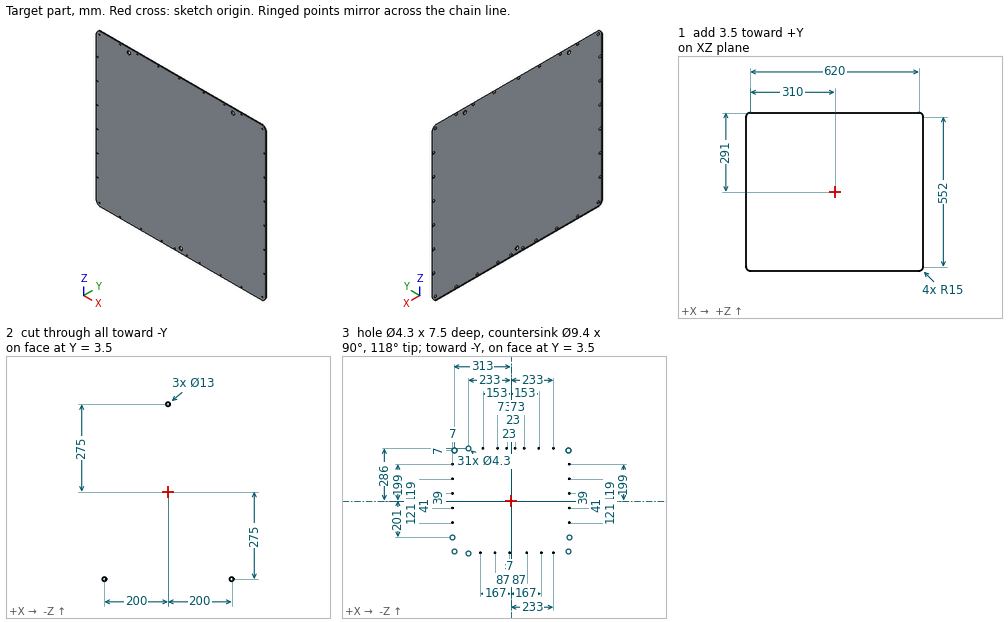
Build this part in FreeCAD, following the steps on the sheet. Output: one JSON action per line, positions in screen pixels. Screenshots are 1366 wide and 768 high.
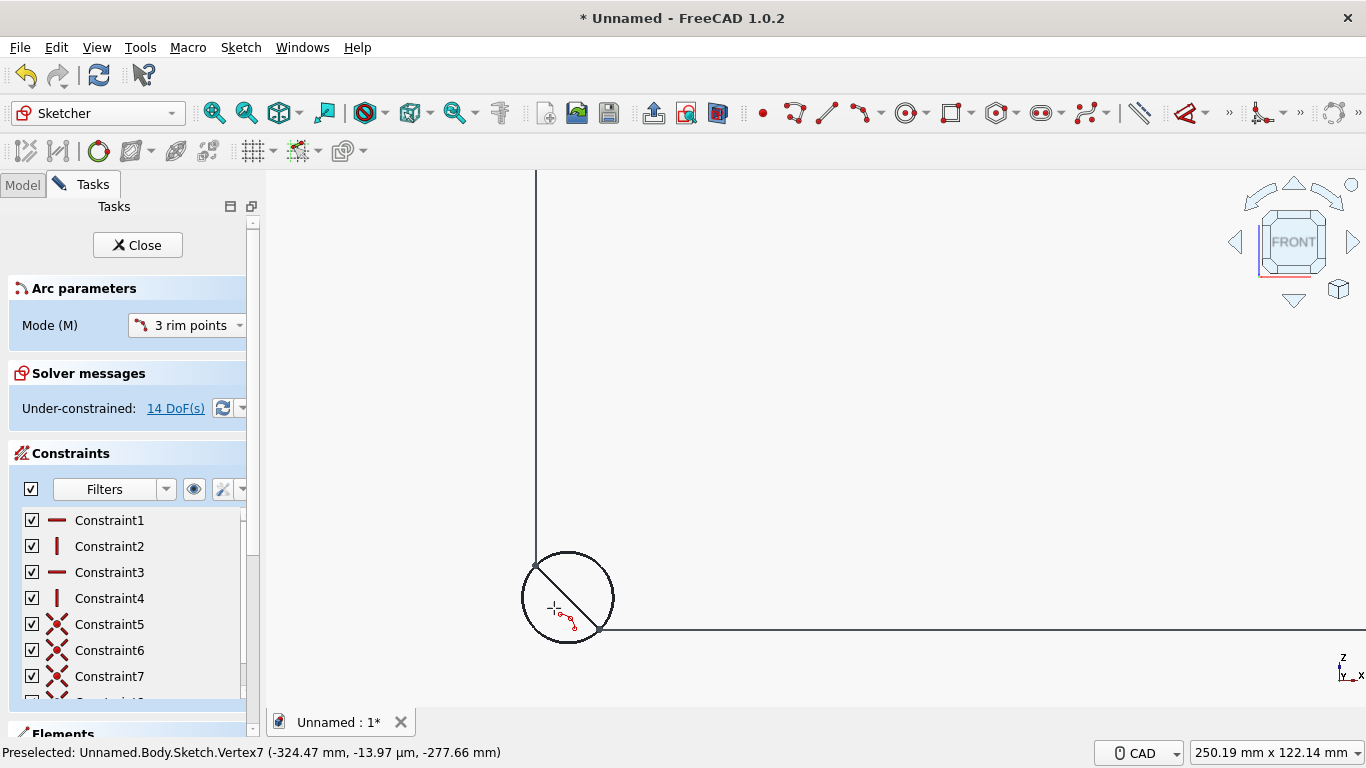
{"action": "left_click", "coordinate": [553, 605]}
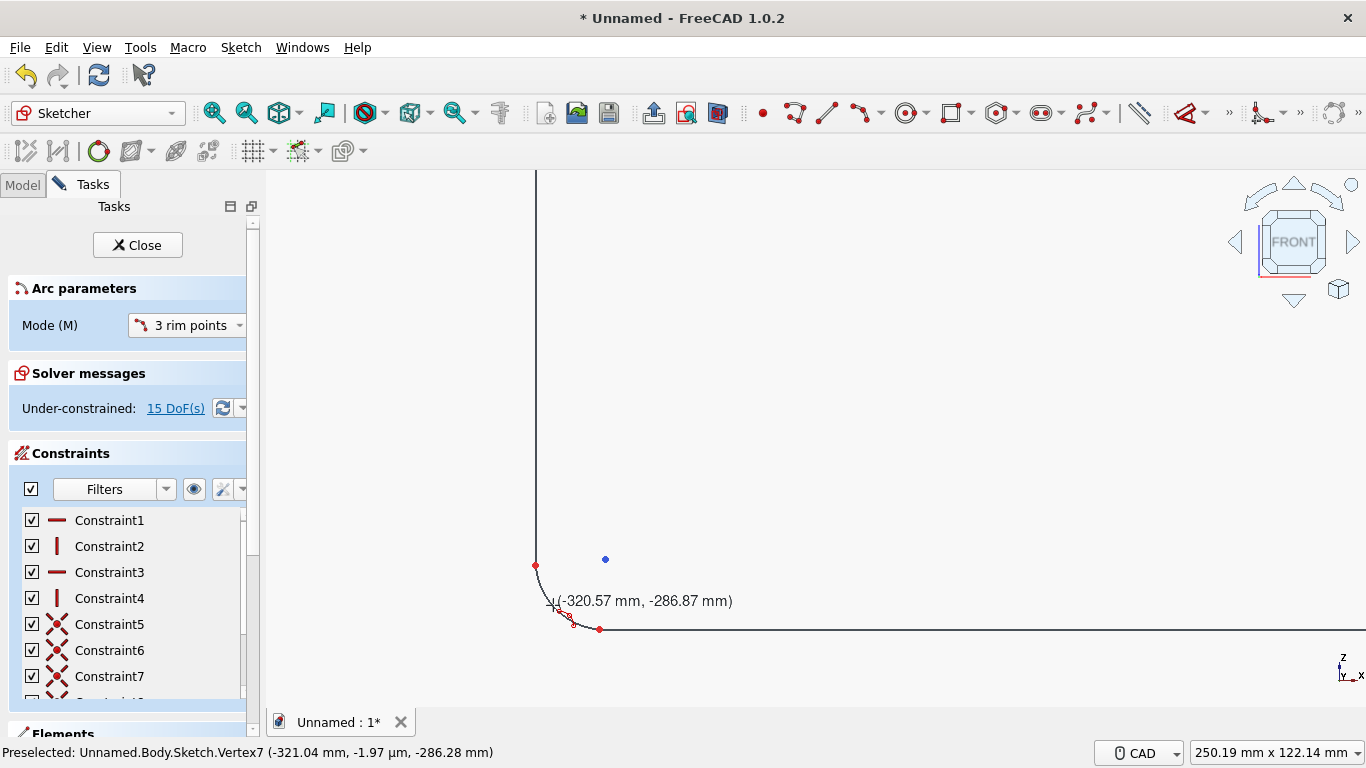
{"action": "scroll", "coordinate": [557, 610], "scroll_direction": "down", "scroll_amount": 10}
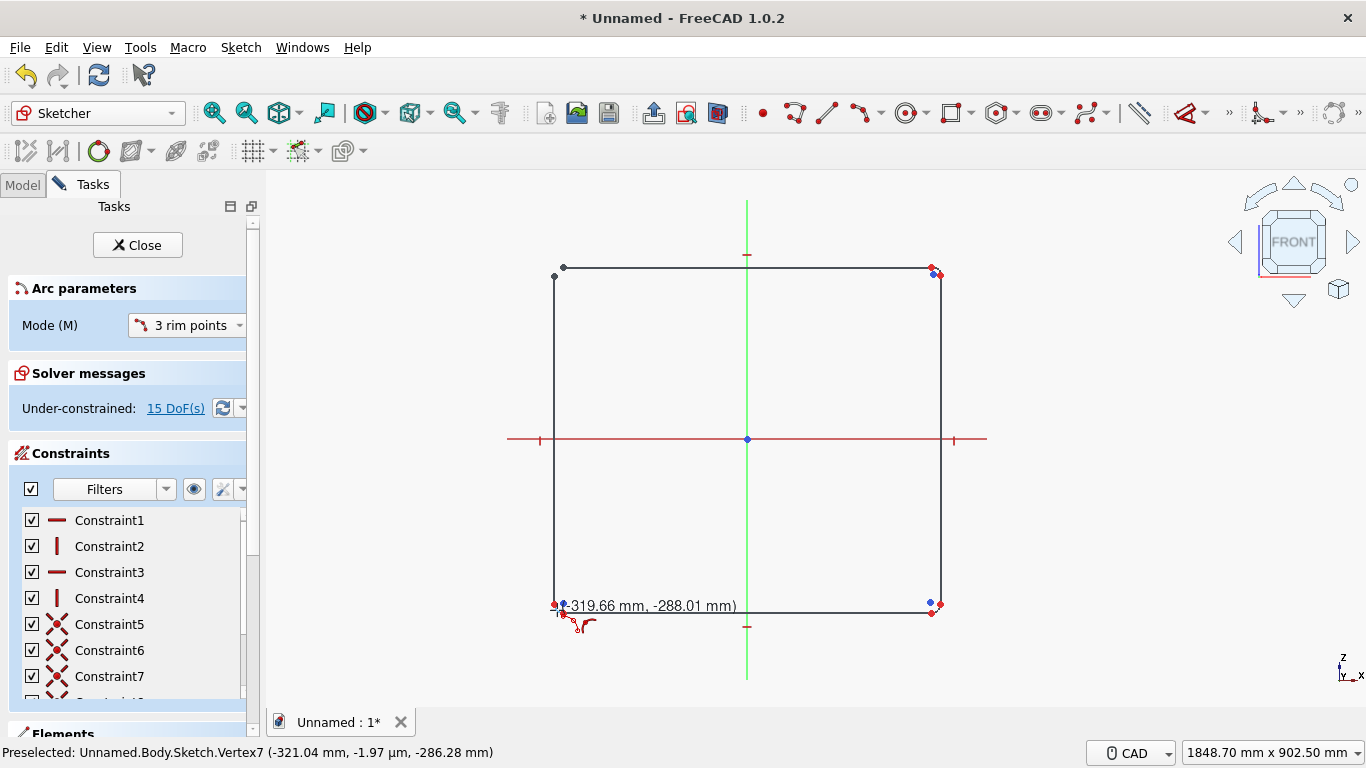
{"action": "scroll", "coordinate": [554, 275], "scroll_direction": "up", "scroll_amount": 2}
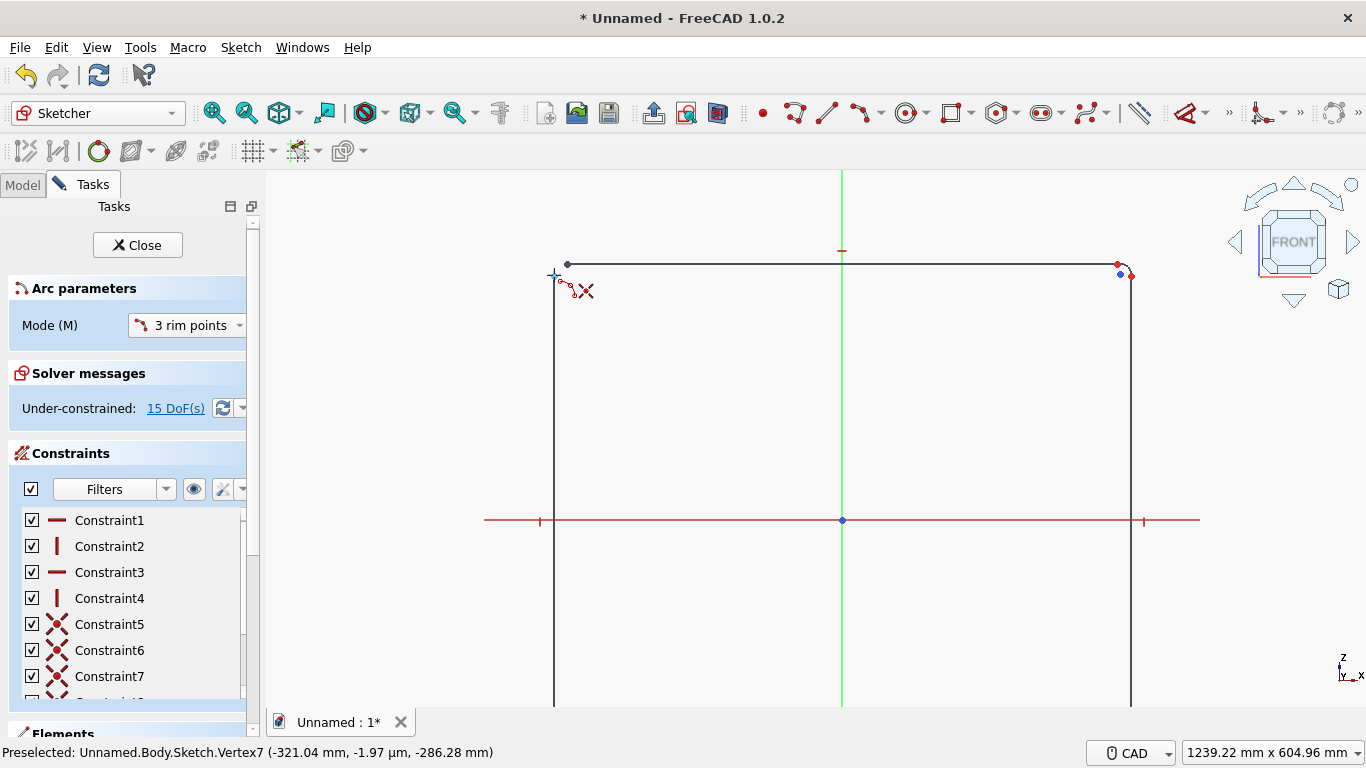
{"action": "left_click", "coordinate": [554, 277]}
{"action": "left_click", "coordinate": [568, 264]}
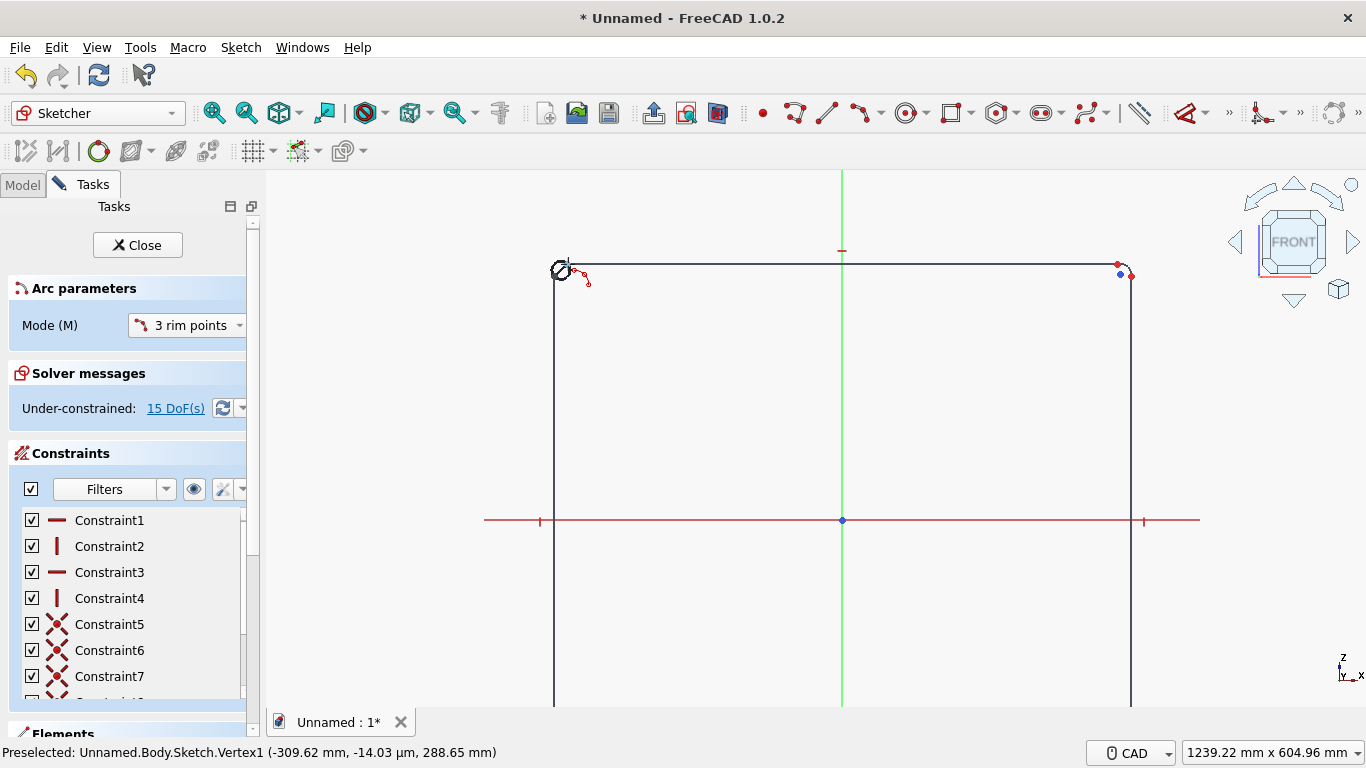
{"action": "scroll", "coordinate": [558, 266], "scroll_direction": "up", "scroll_amount": 8}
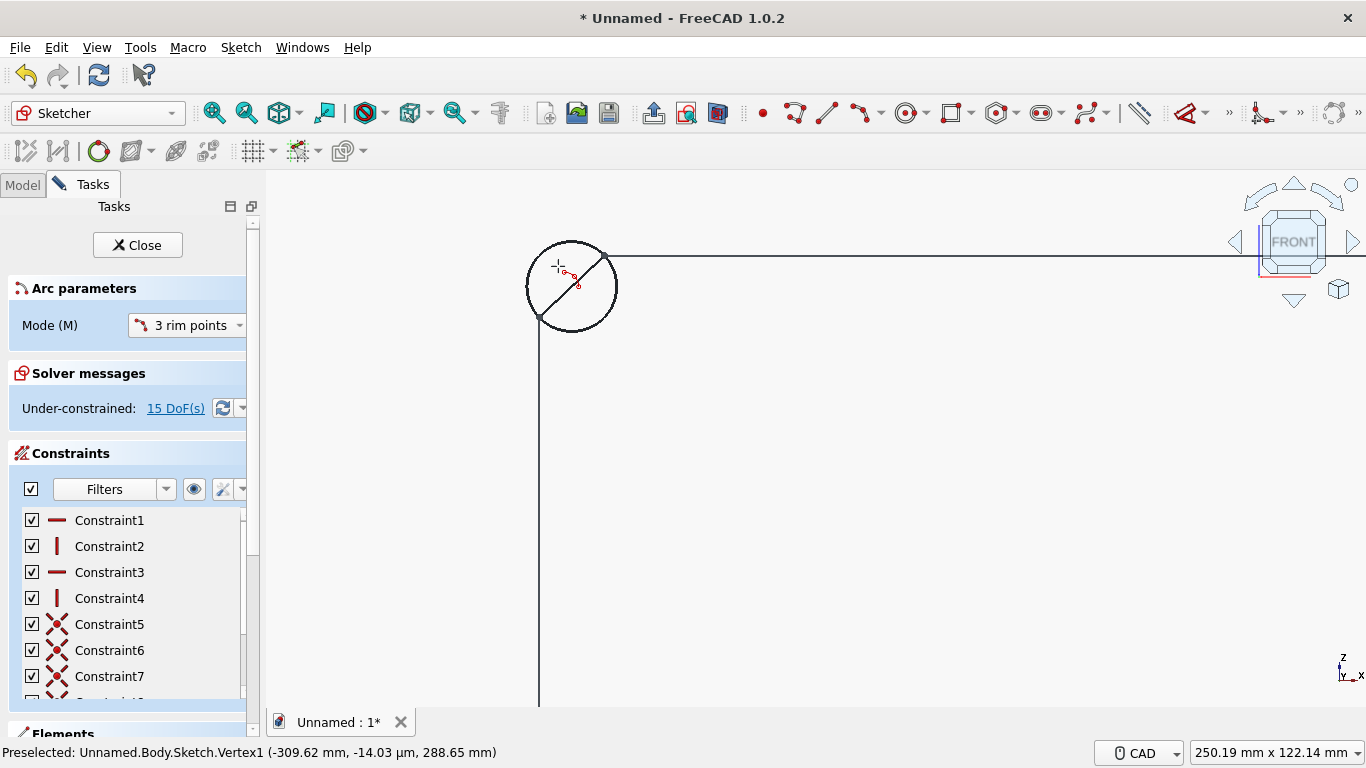
{"action": "left_click", "coordinate": [556, 265]}
{"action": "key", "text": "Escape"}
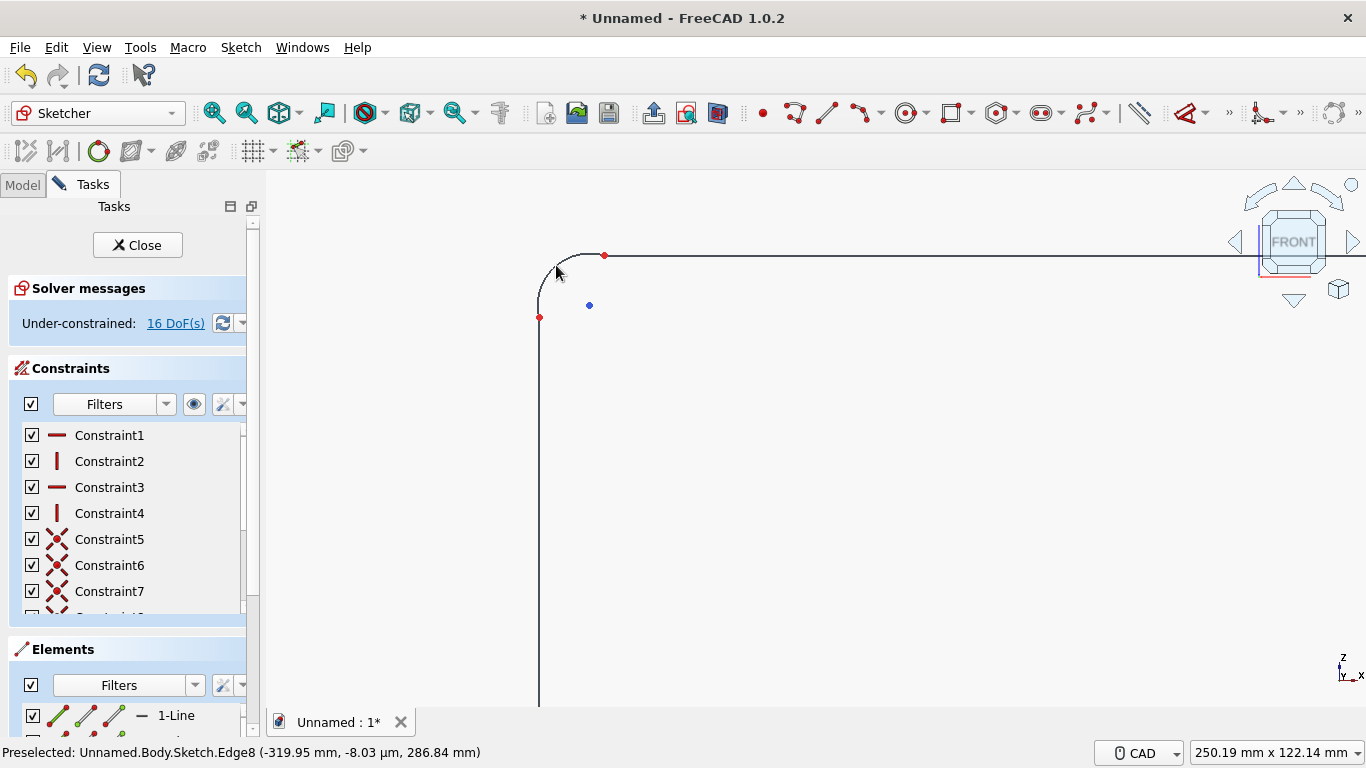
{"action": "scroll", "coordinate": [557, 268], "scroll_direction": "down", "scroll_amount": 10}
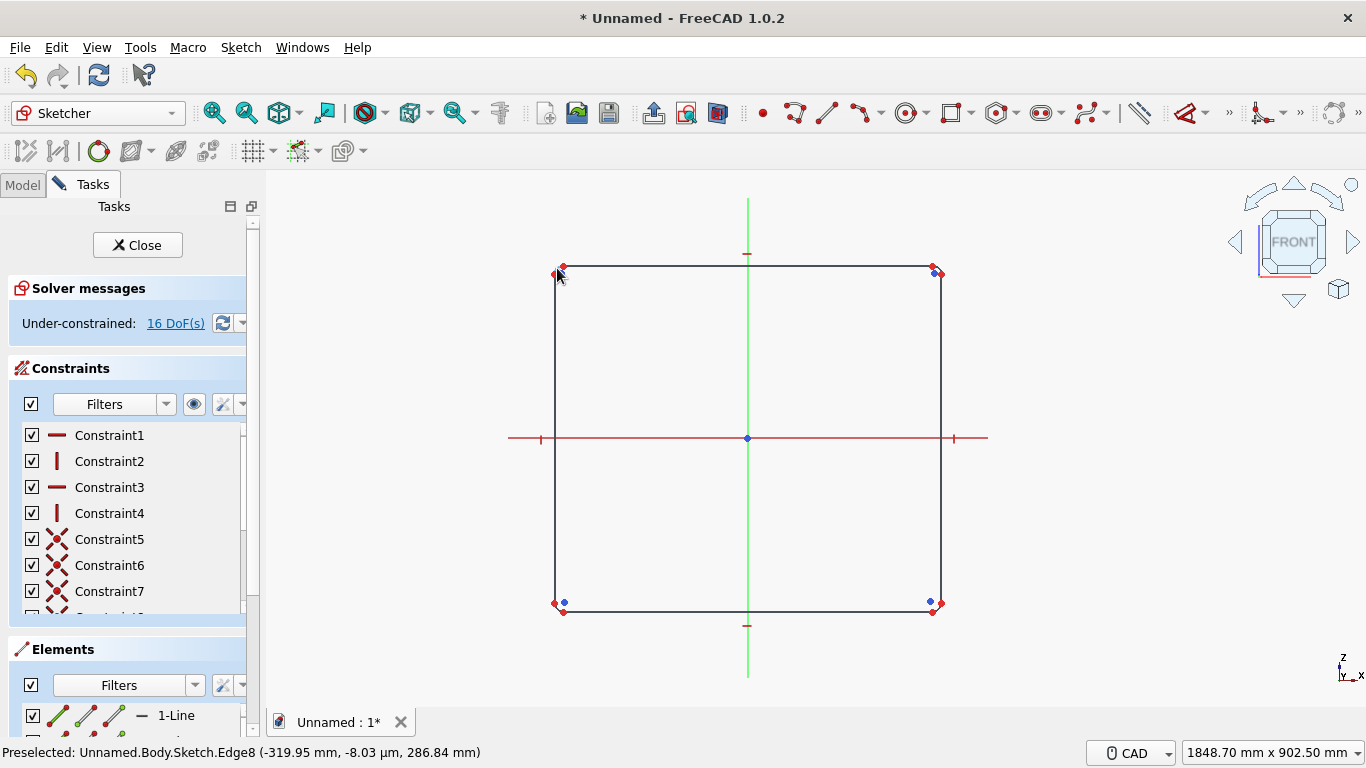
{"action": "left_click", "coordinate": [637, 266]}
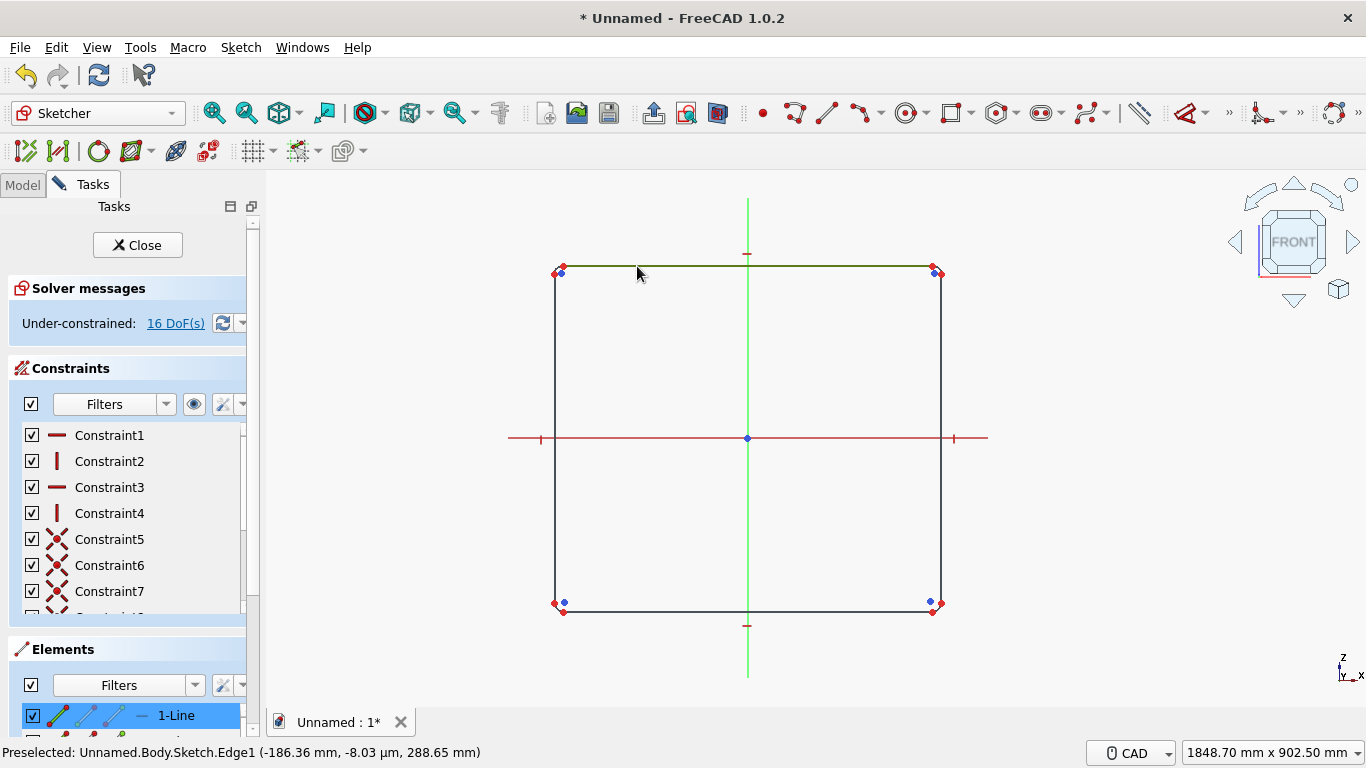
{"action": "scroll", "coordinate": [939, 268], "scroll_direction": "up", "scroll_amount": 4}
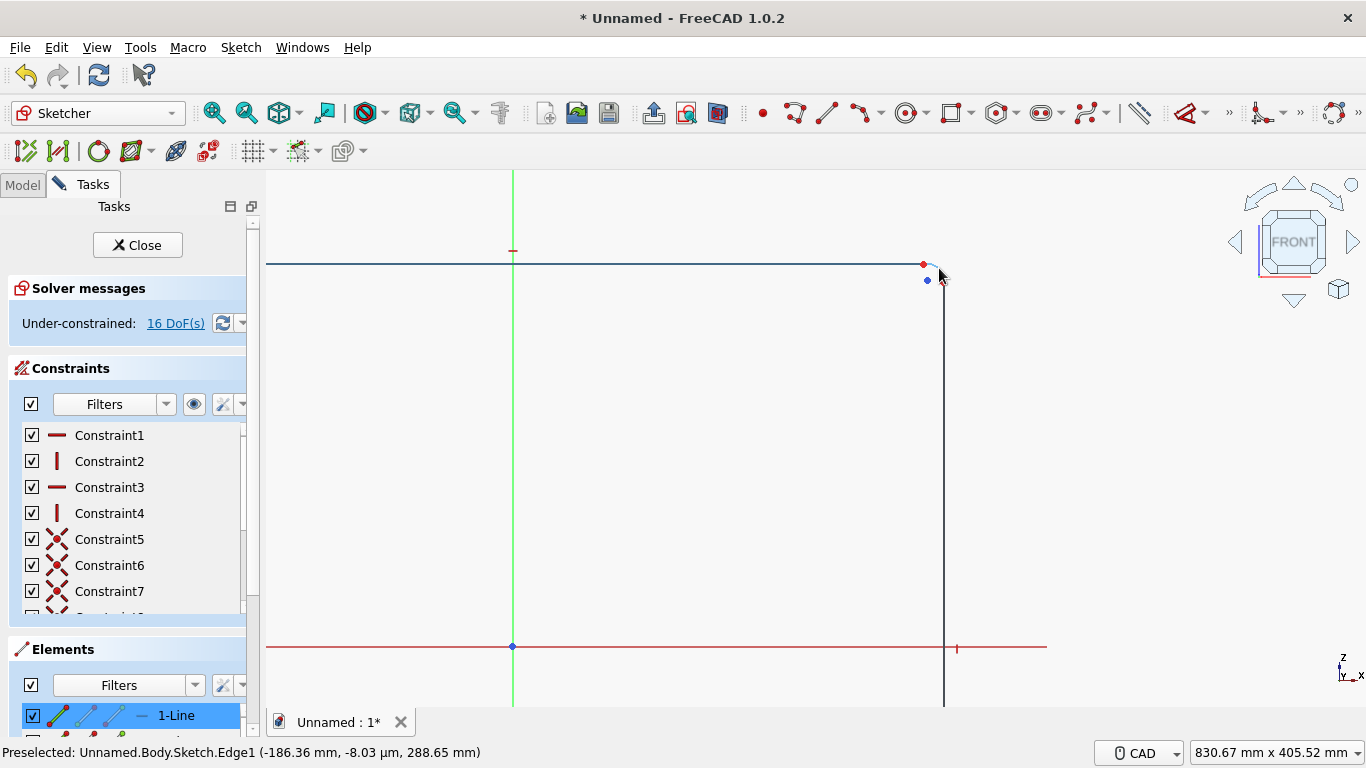
{"action": "left_click", "coordinate": [938, 268]}